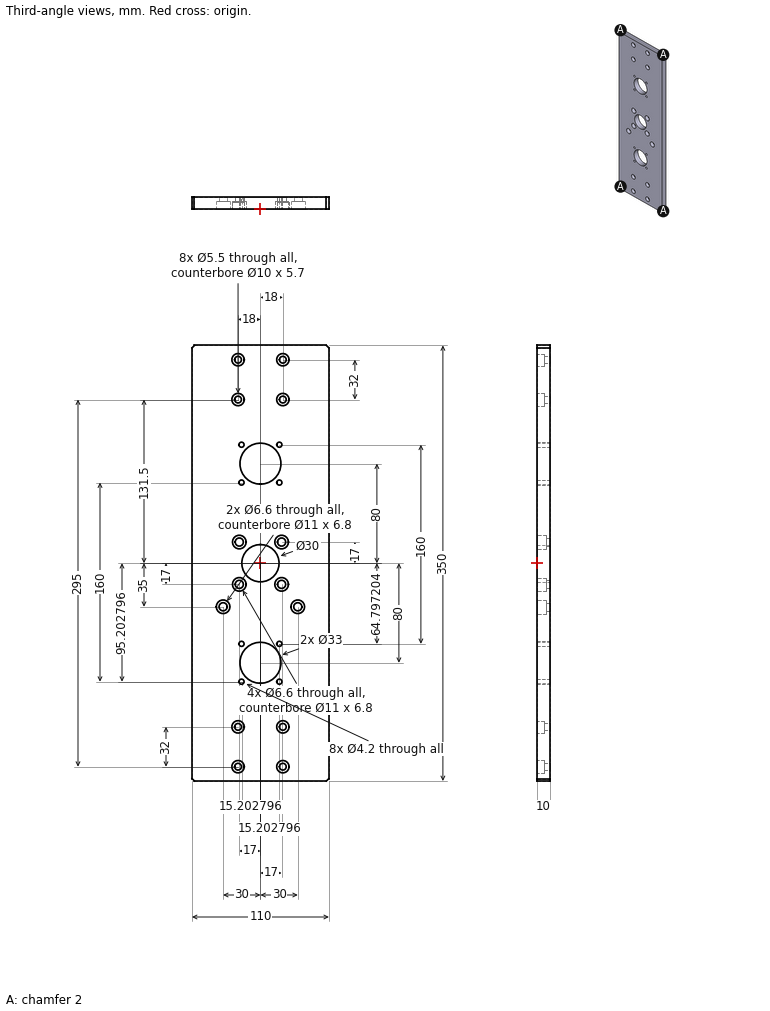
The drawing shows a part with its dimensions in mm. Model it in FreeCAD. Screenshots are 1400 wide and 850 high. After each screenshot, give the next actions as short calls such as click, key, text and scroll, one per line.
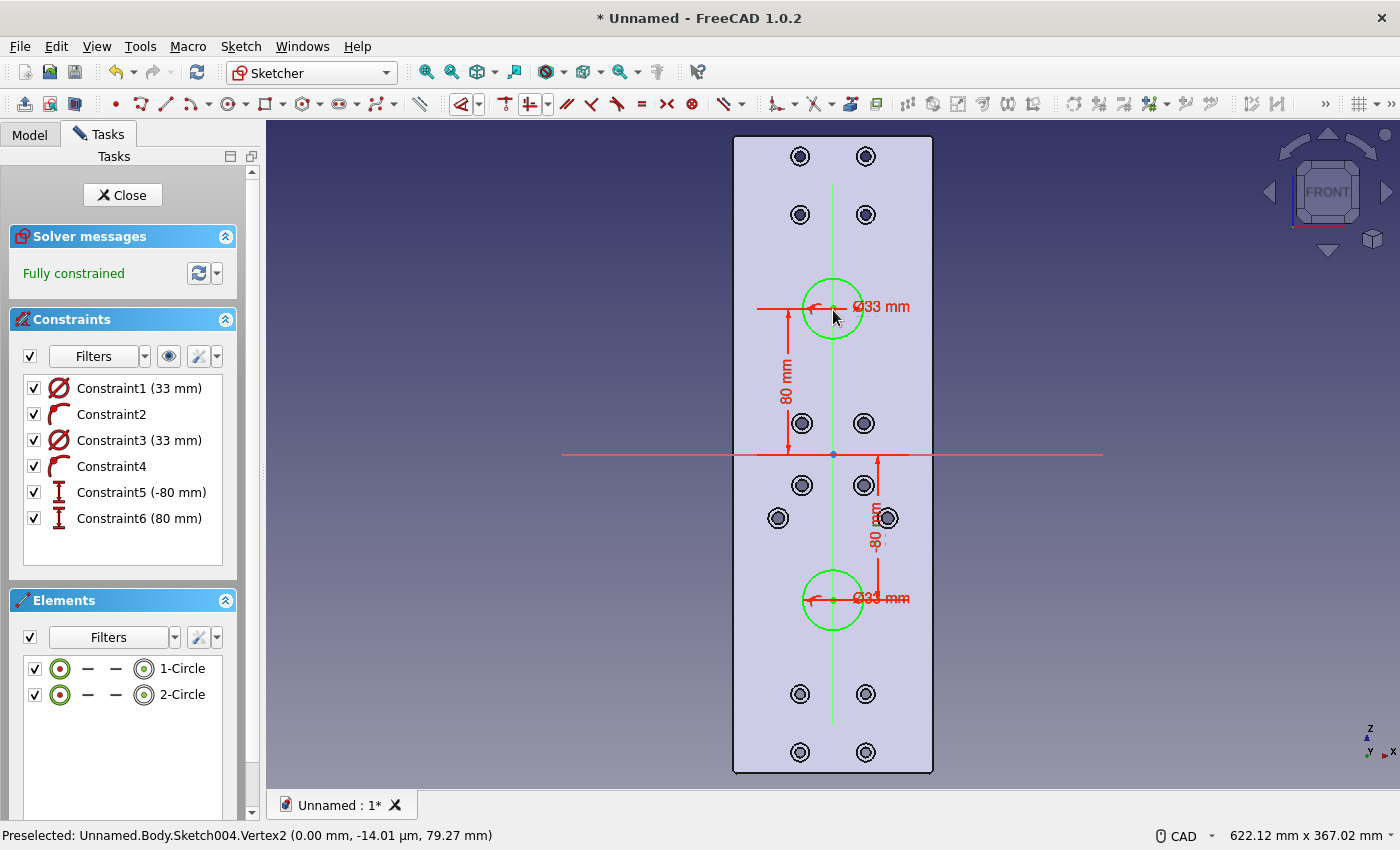
click(123, 195)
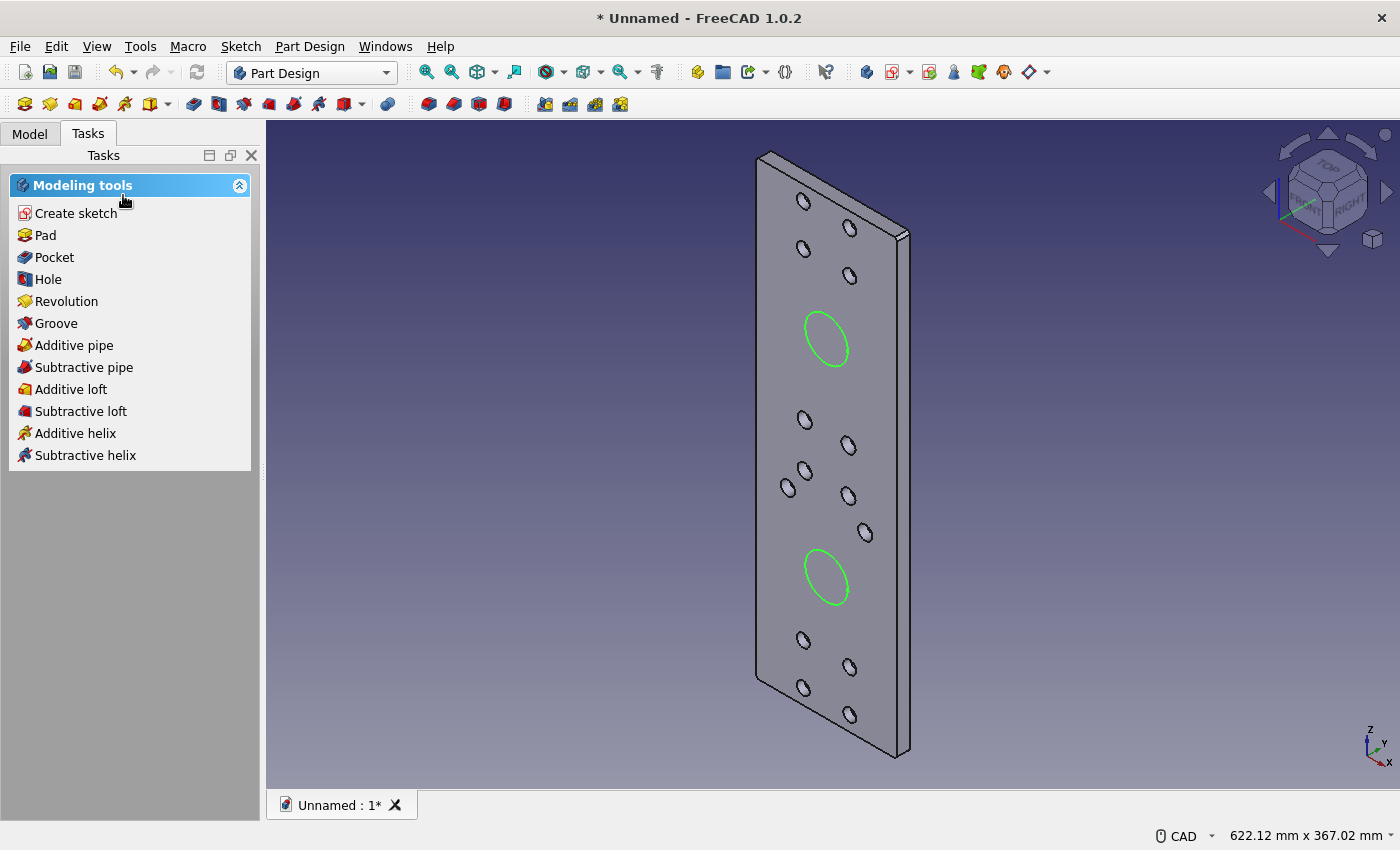
click(194, 104)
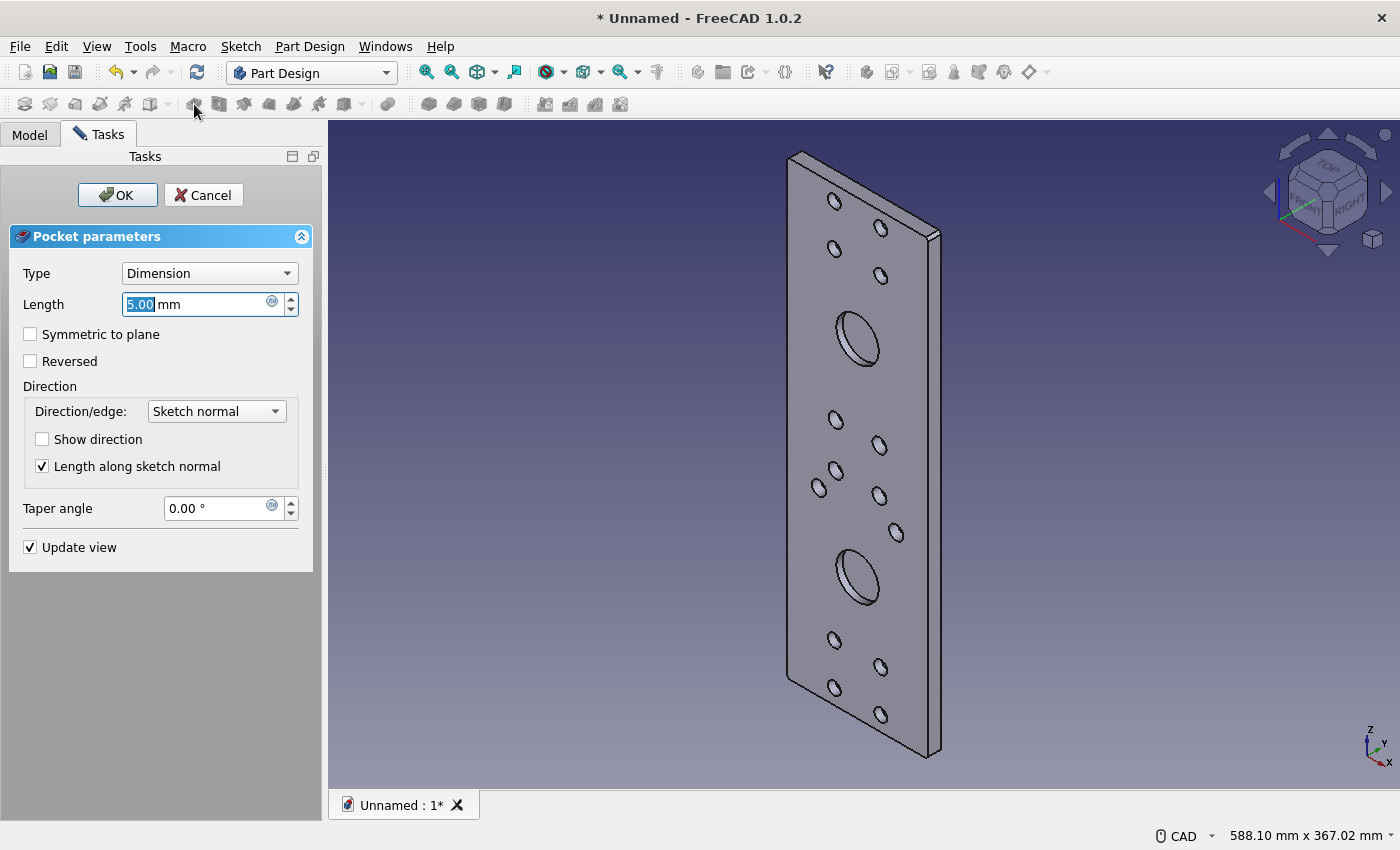
click(210, 274)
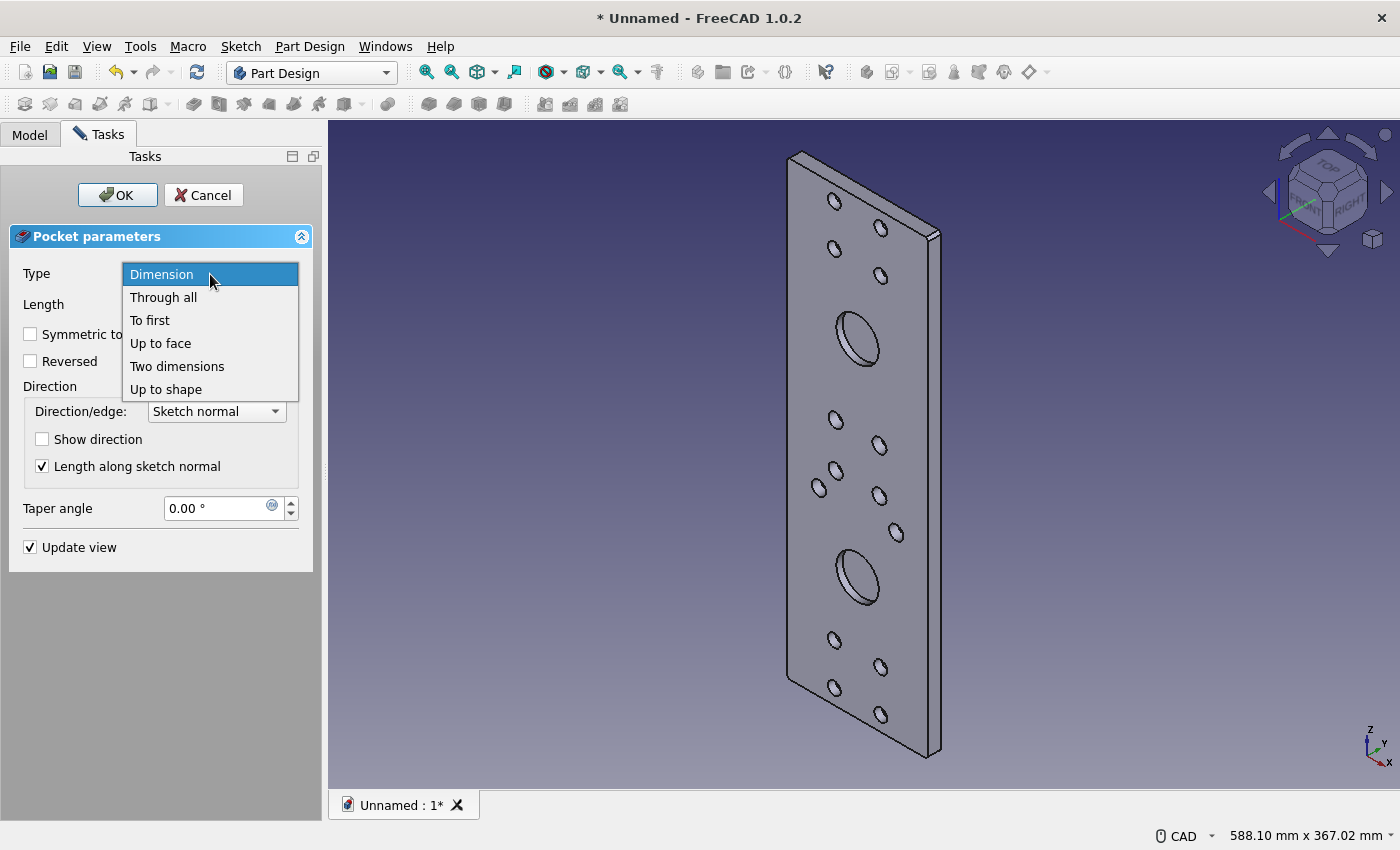
click(208, 298)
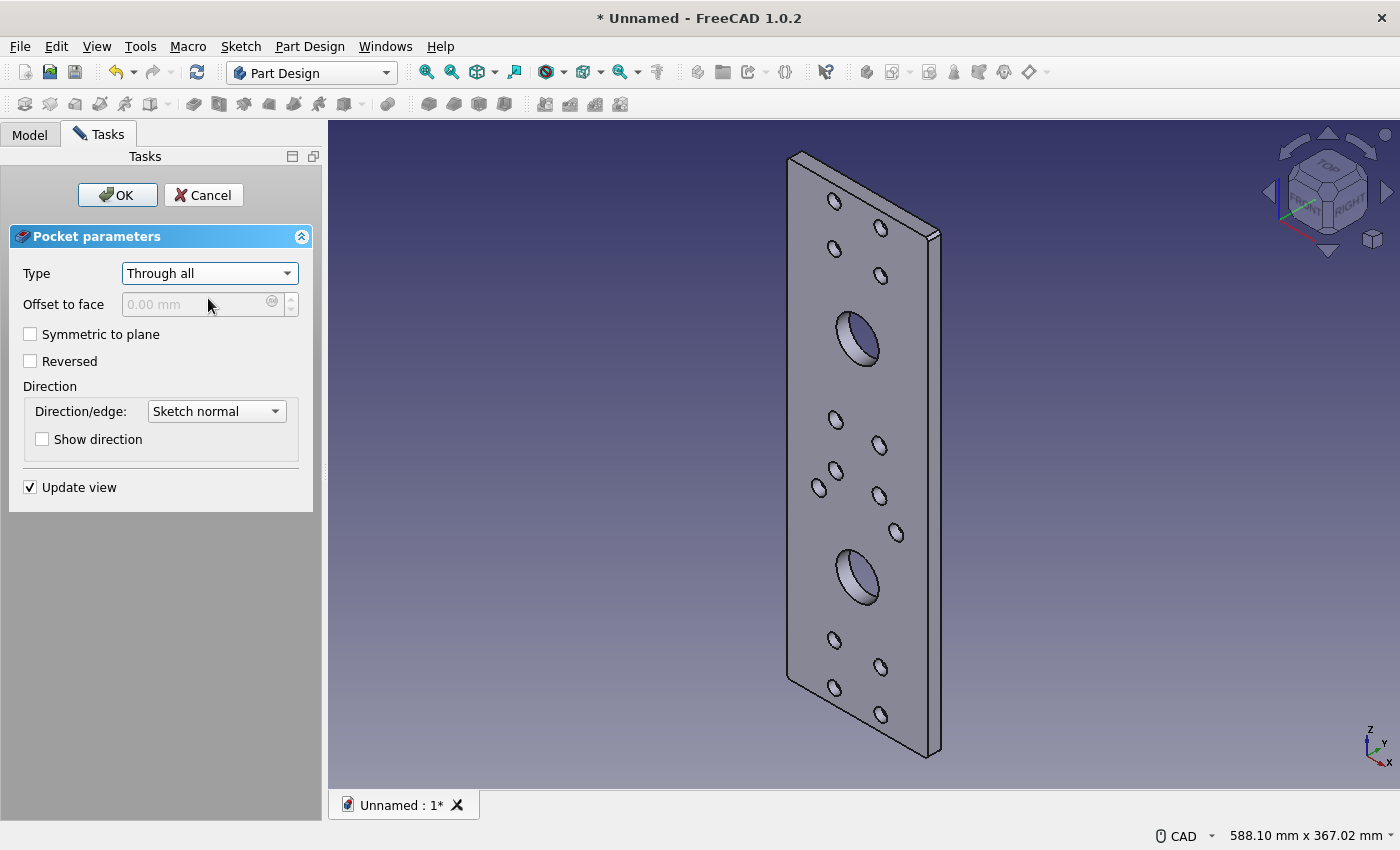
click(118, 195)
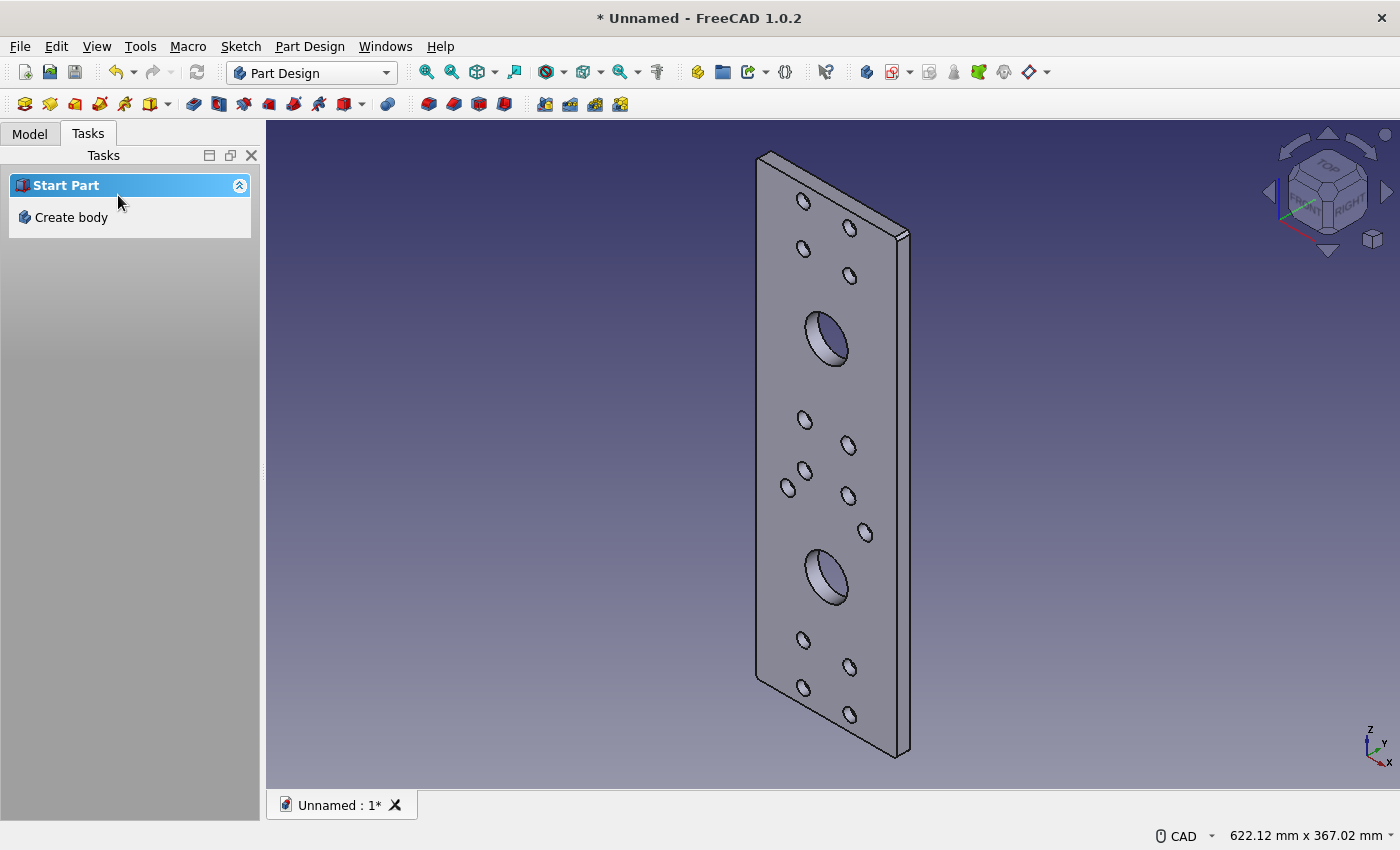
key(4)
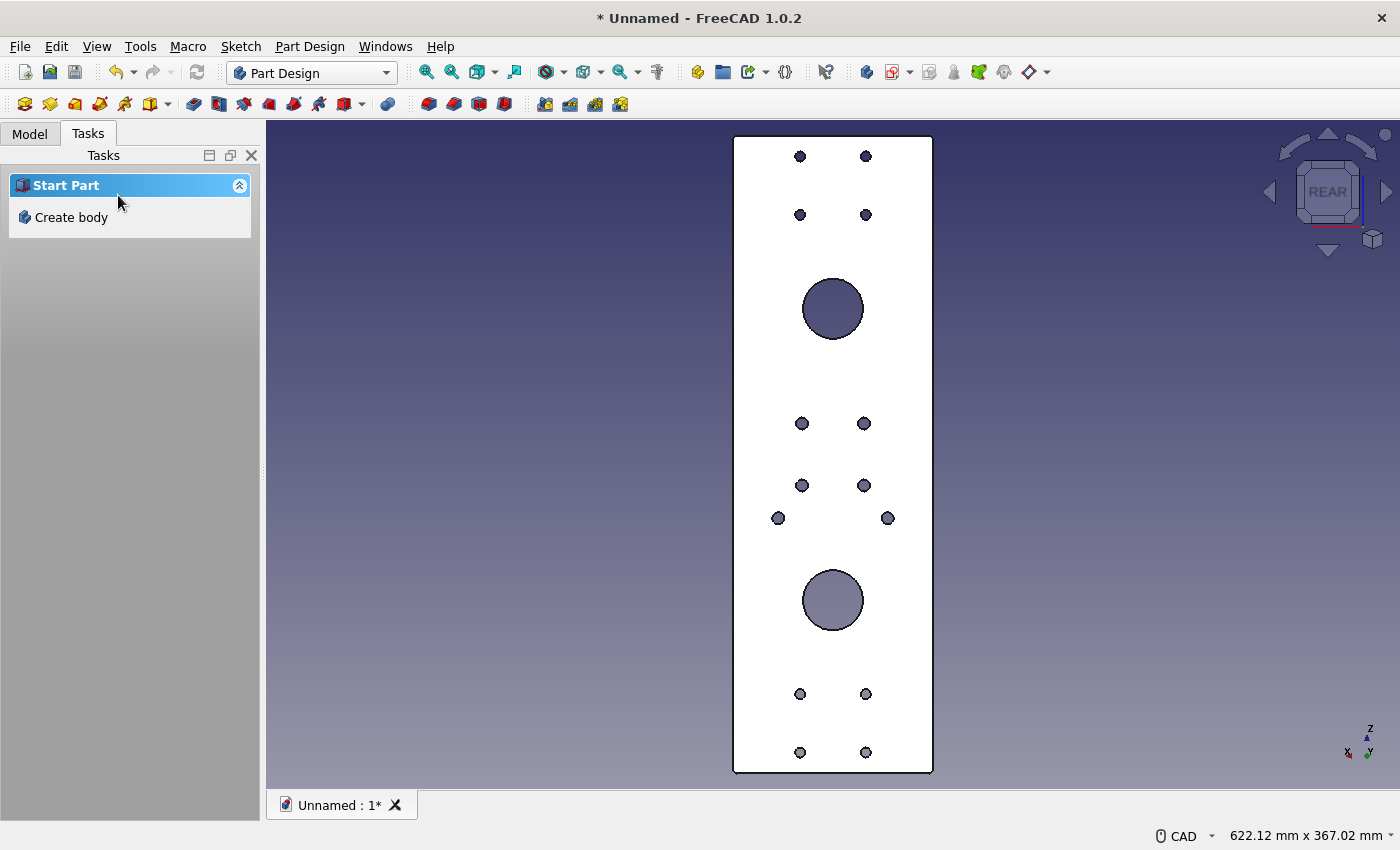
click(890, 362)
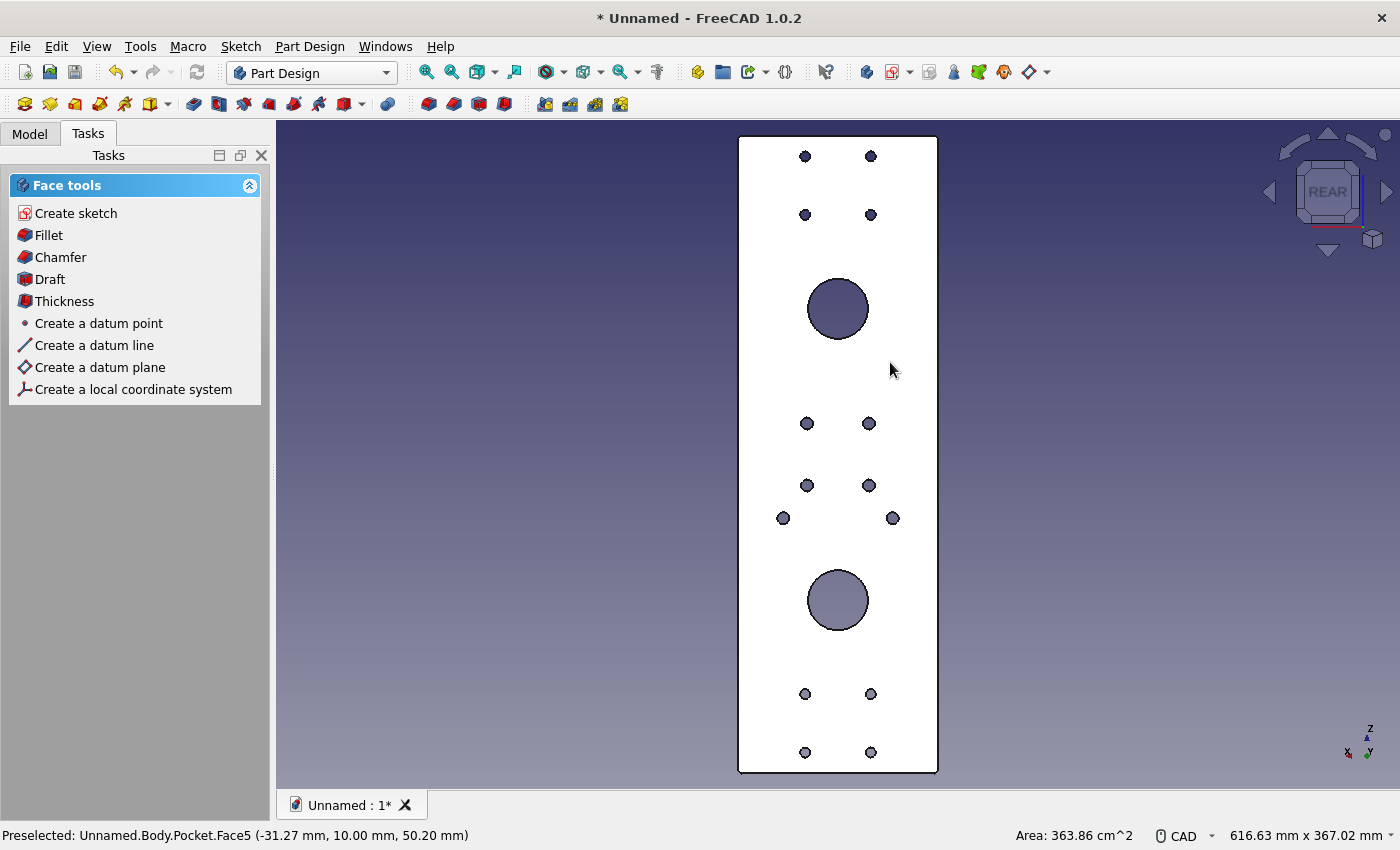
click(892, 72)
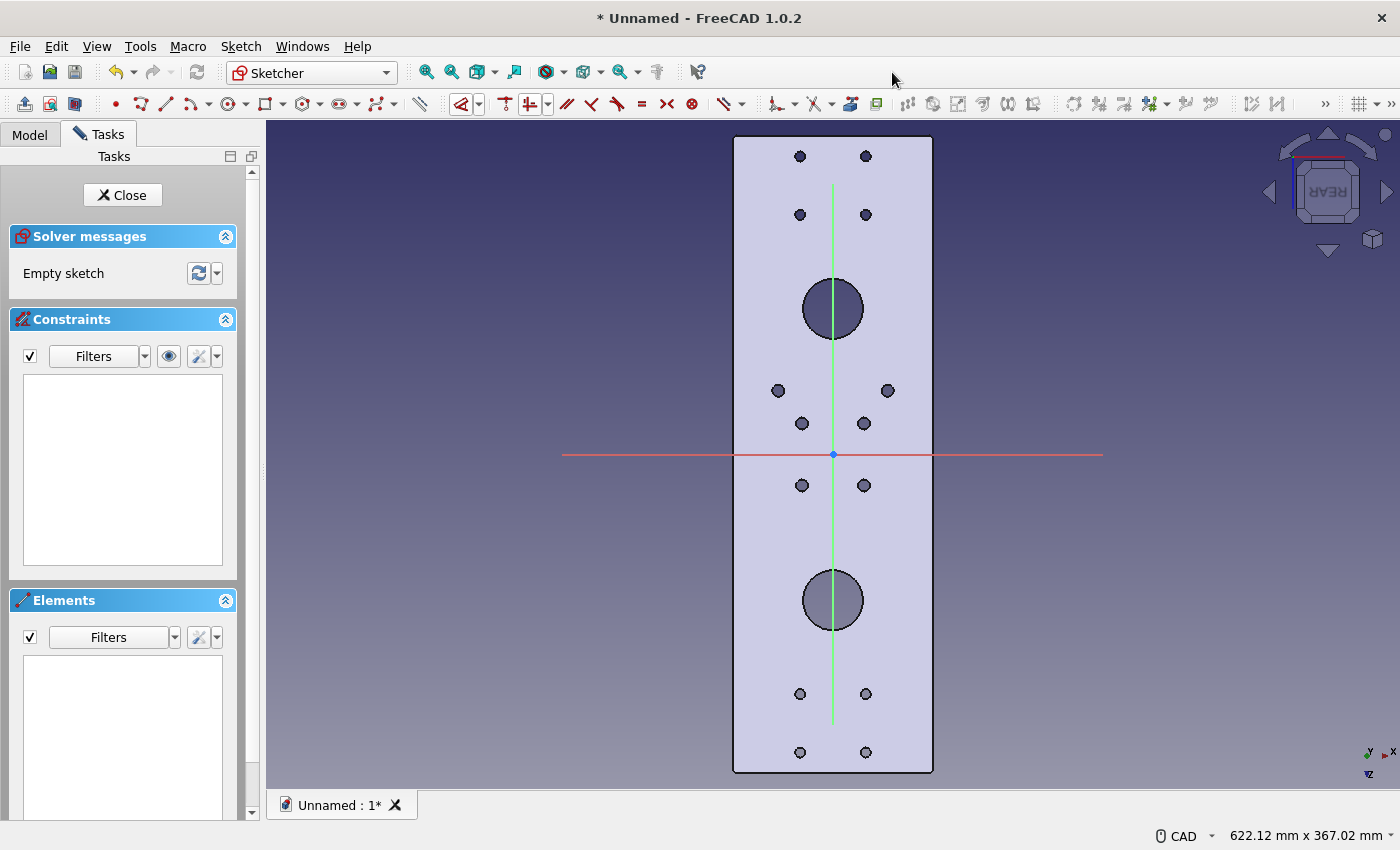
key(g)
key(c)